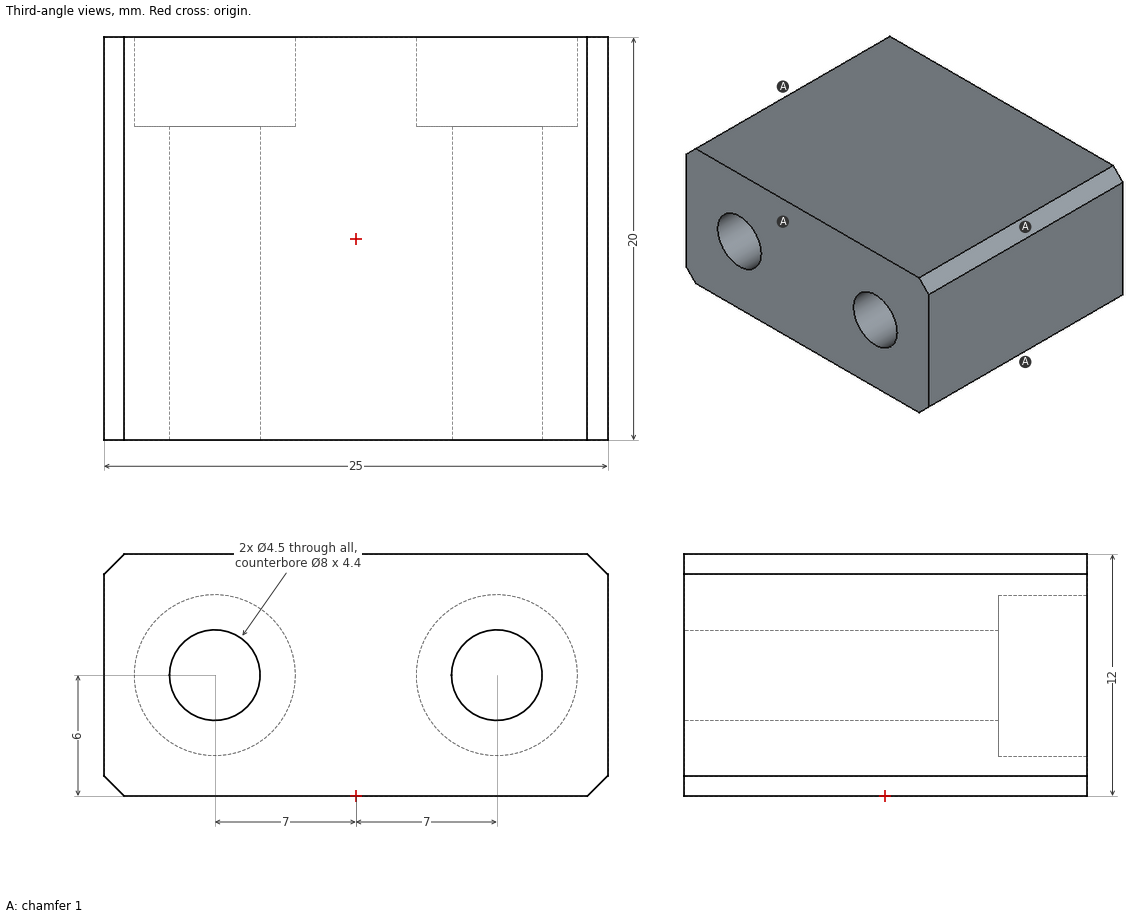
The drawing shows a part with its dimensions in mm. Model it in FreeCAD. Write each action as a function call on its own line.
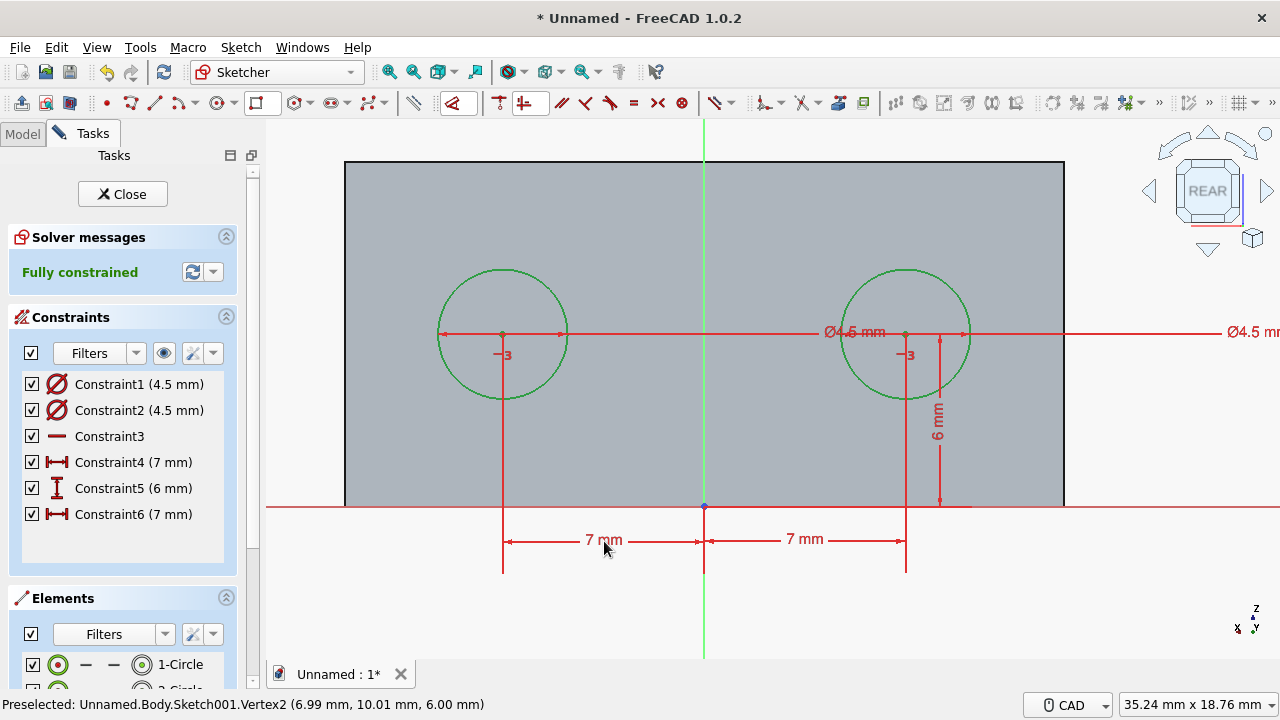
click(123, 194)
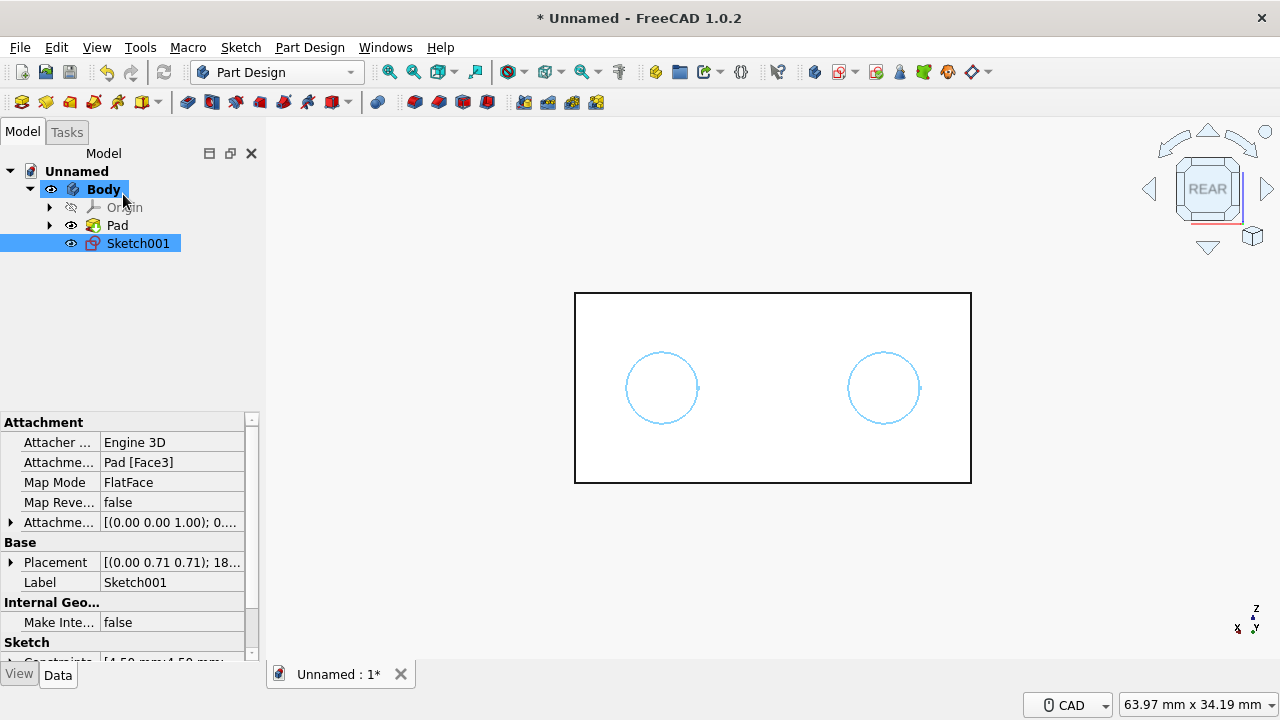
click(212, 102)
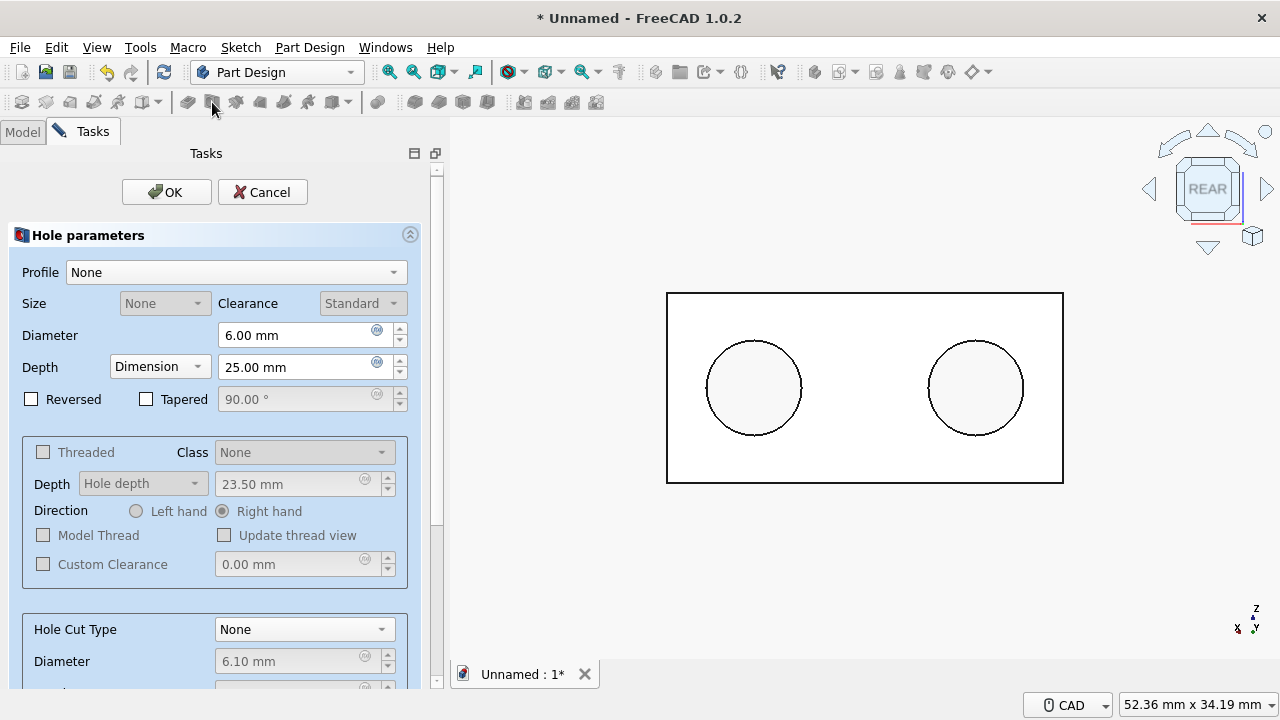
triple_click(305, 335)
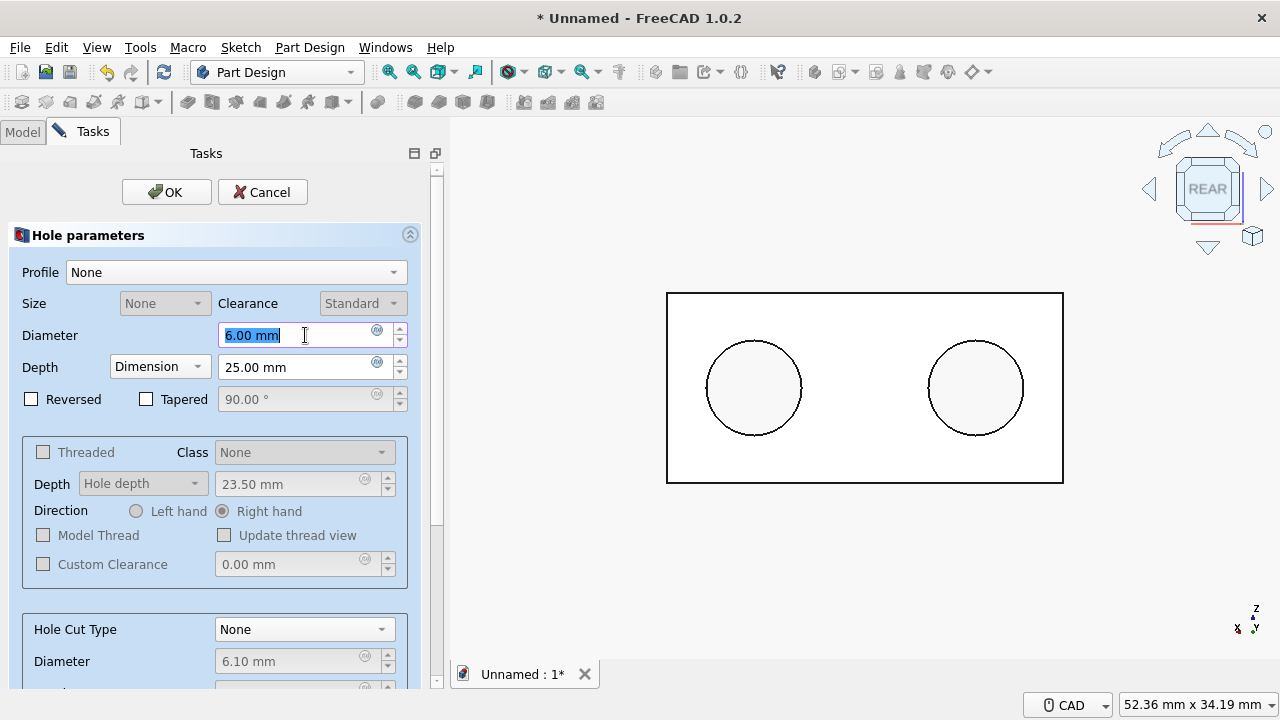
text(4.5)
key(Tab)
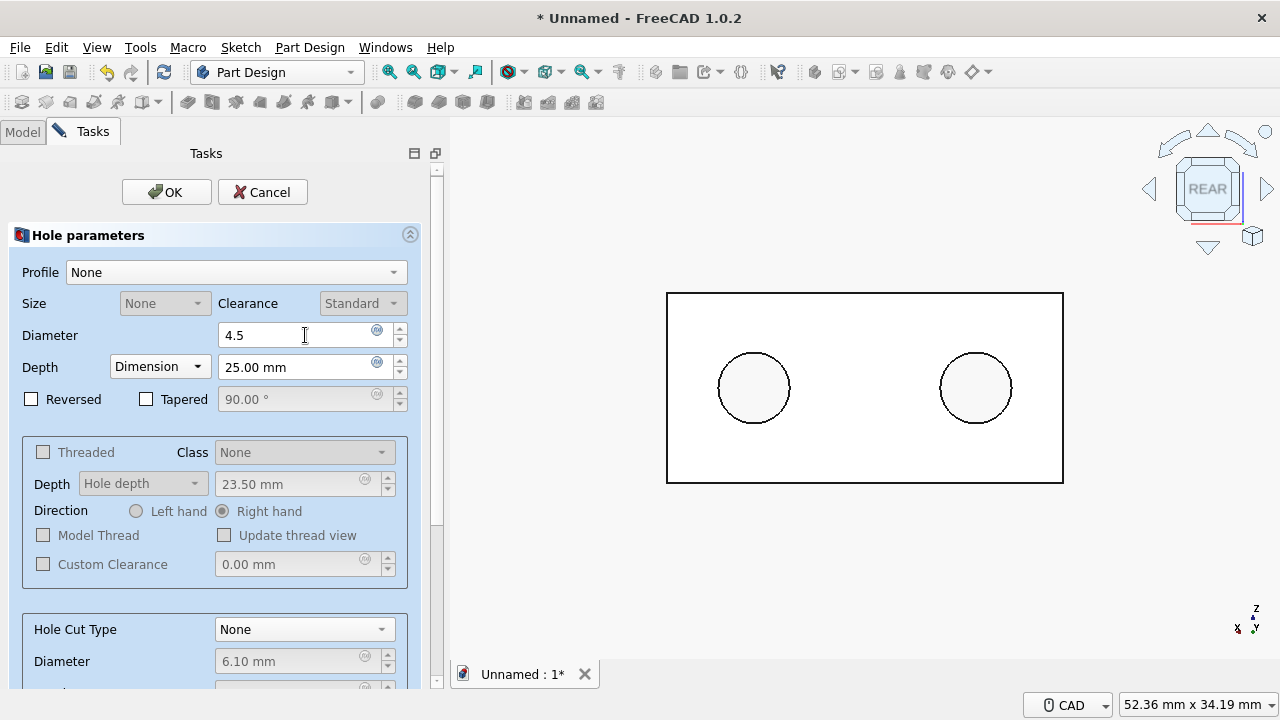
click(161, 366)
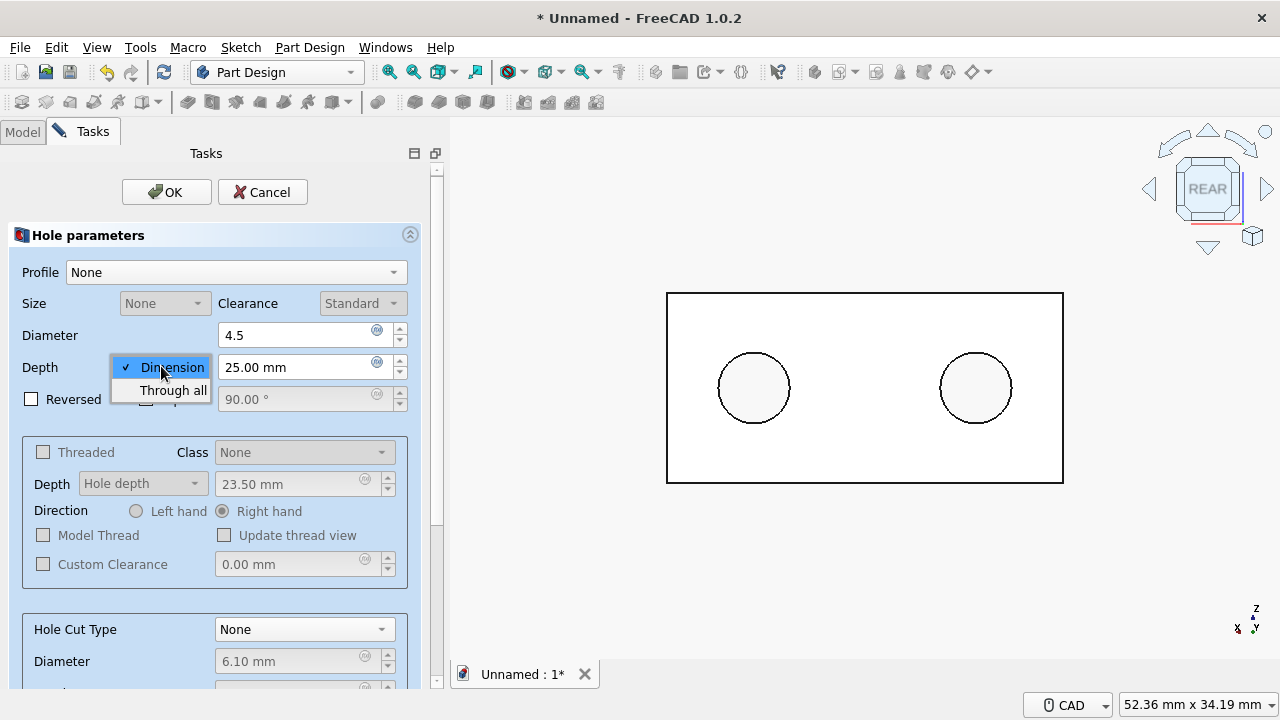
click(160, 390)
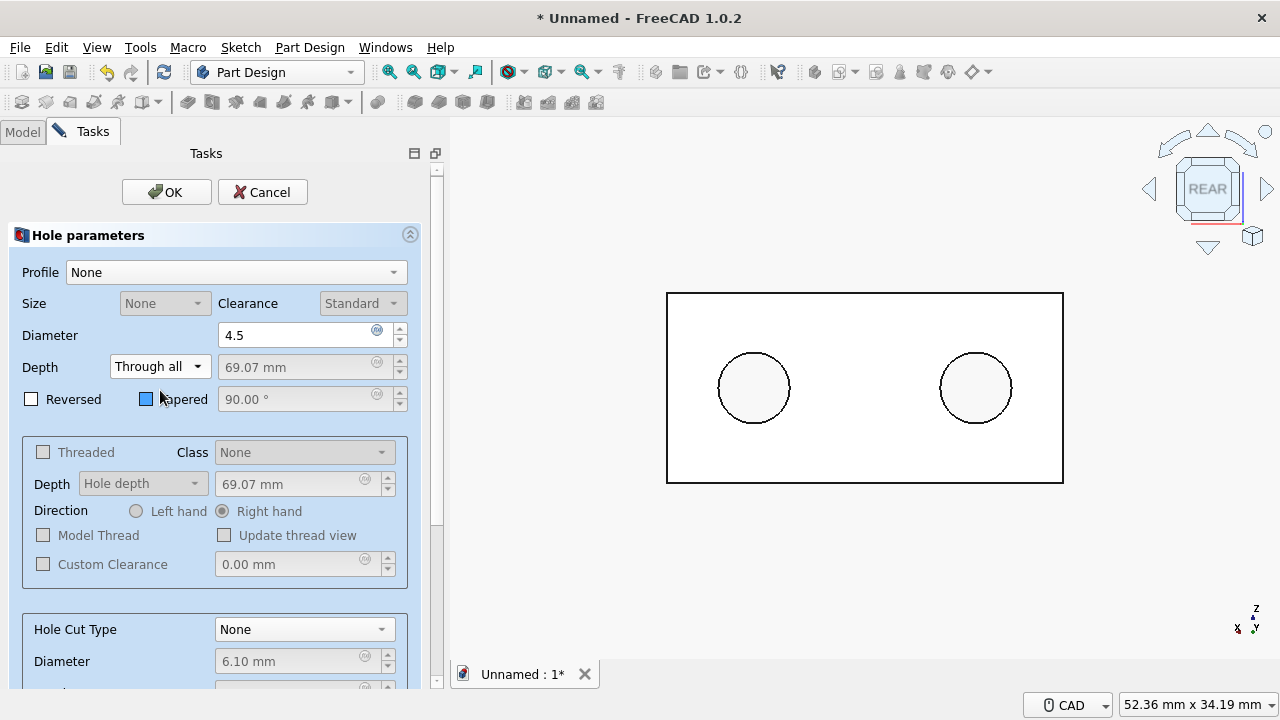
click(306, 630)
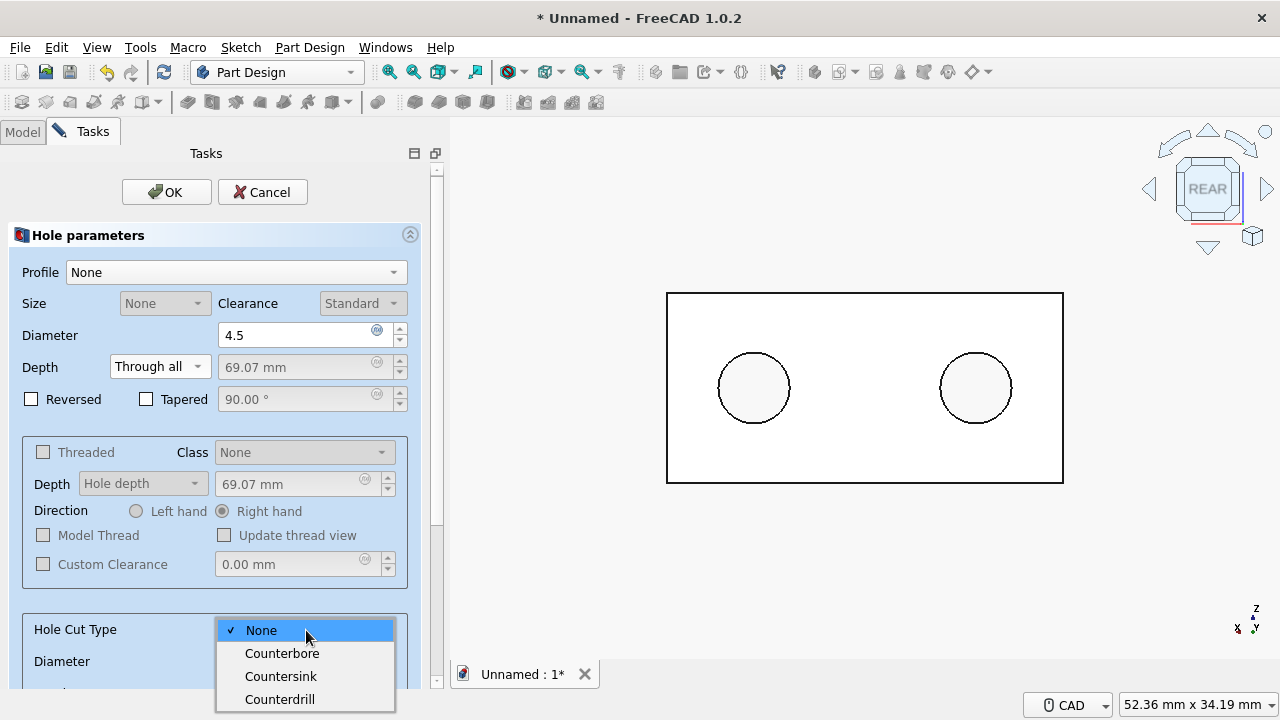
click(304, 654)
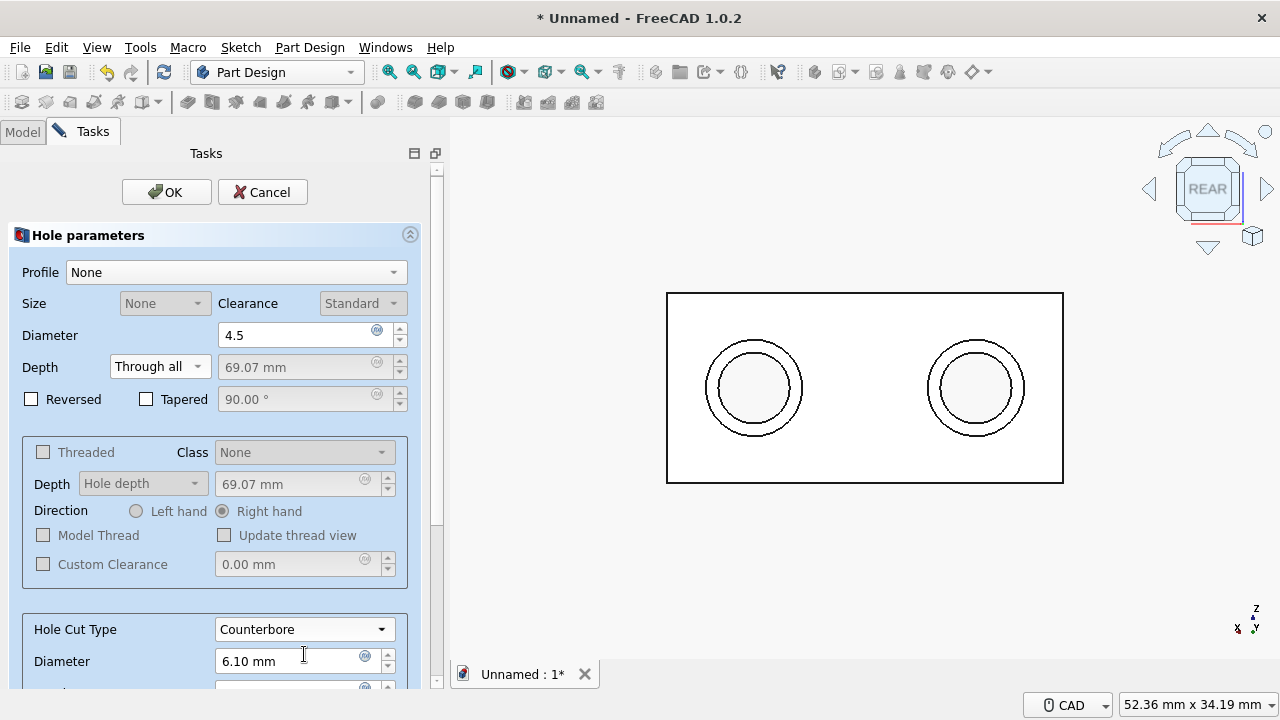
triple_click(298, 661)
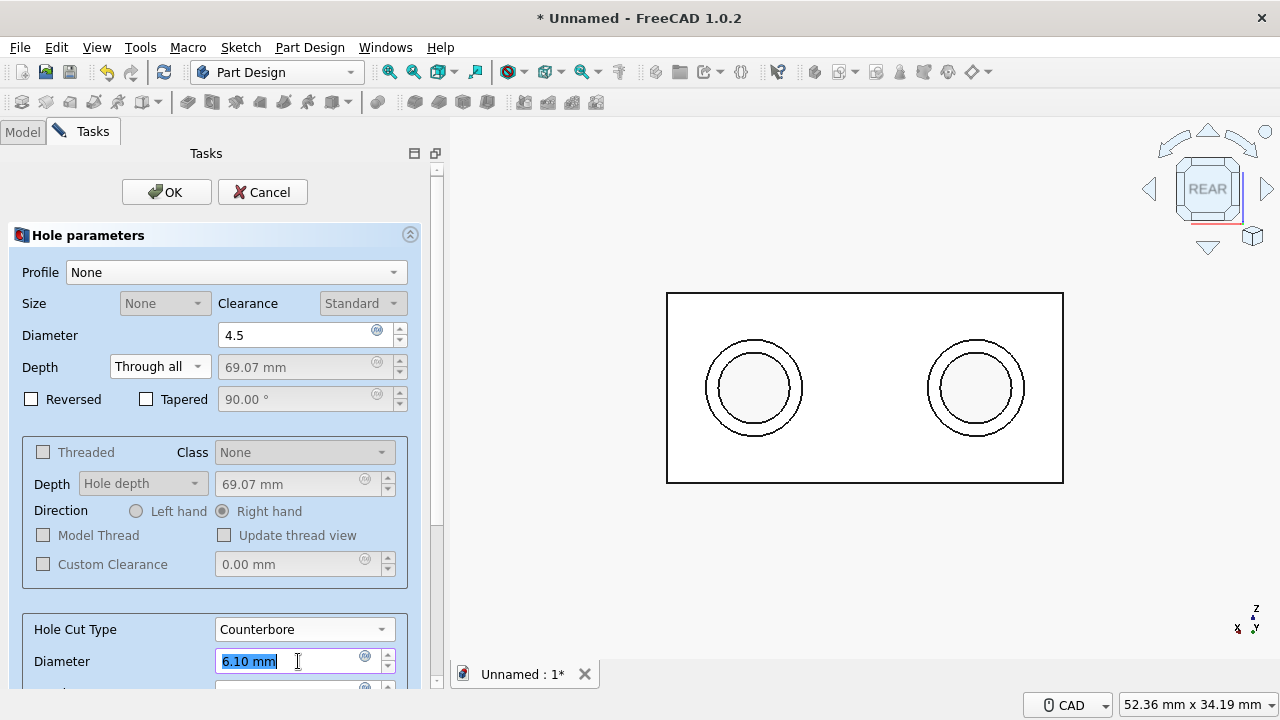
text(8)
key(Tab)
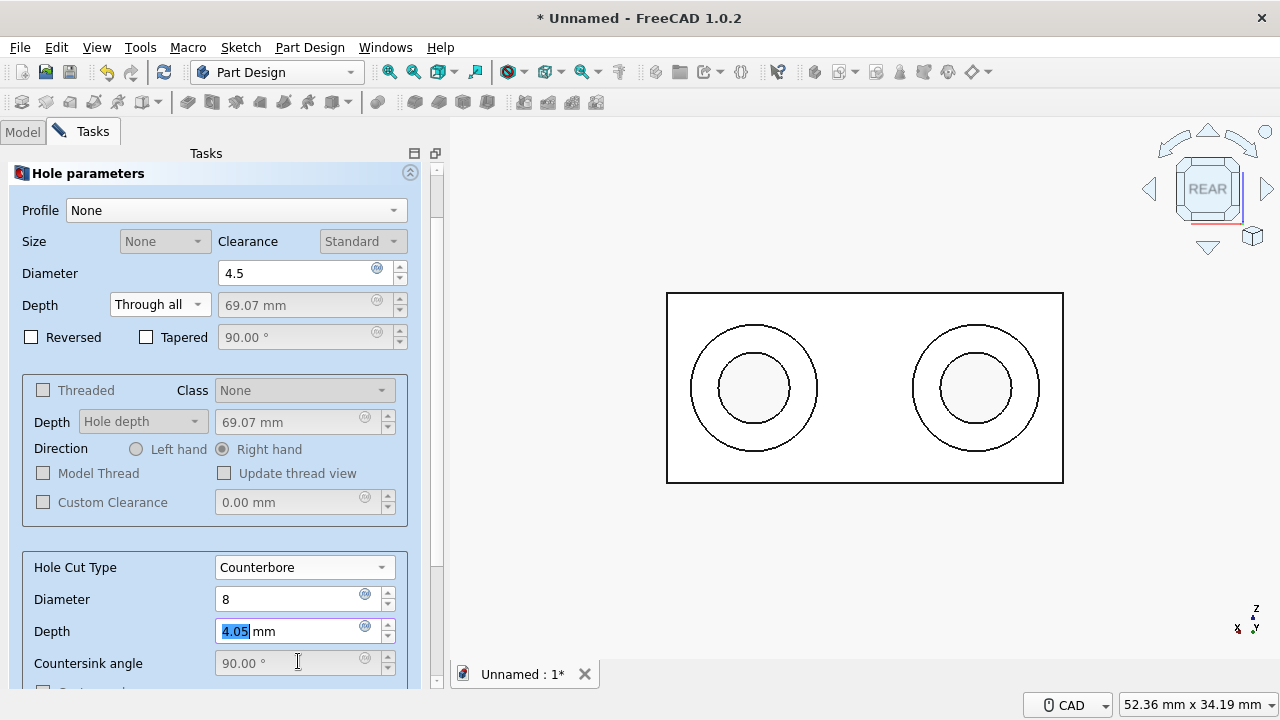
text(4.4)
key(Tab)